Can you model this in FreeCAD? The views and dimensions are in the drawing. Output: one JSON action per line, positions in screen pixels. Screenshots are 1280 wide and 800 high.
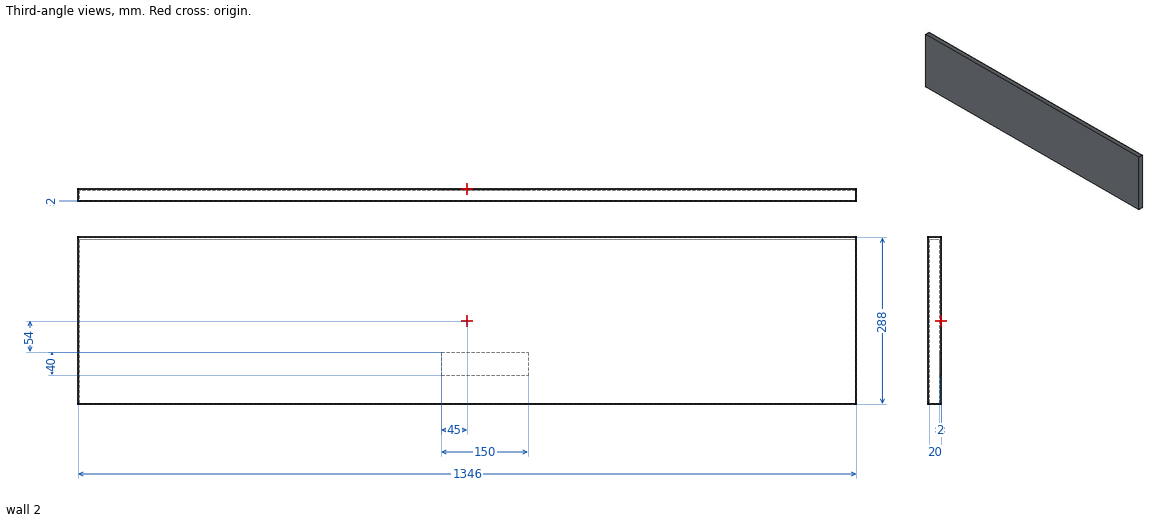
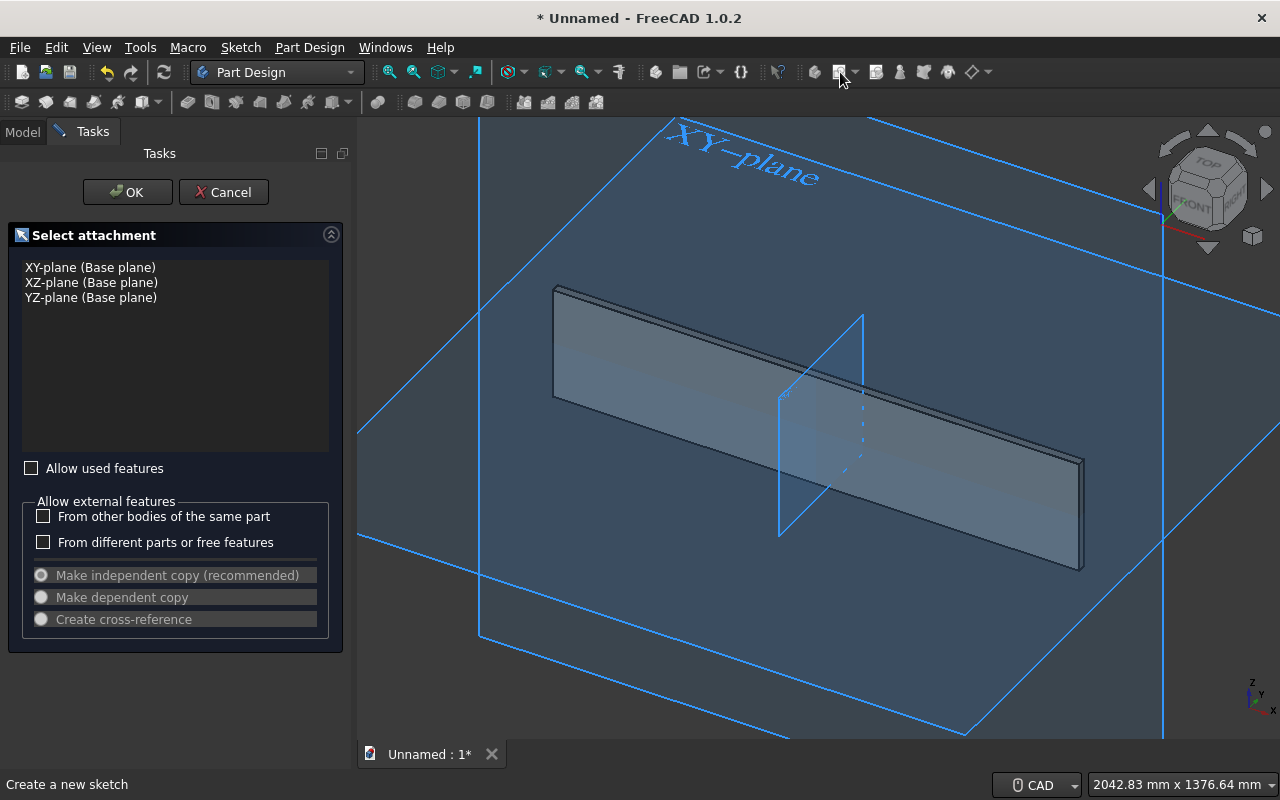
{"action": "left_click", "coordinate": [82, 282]}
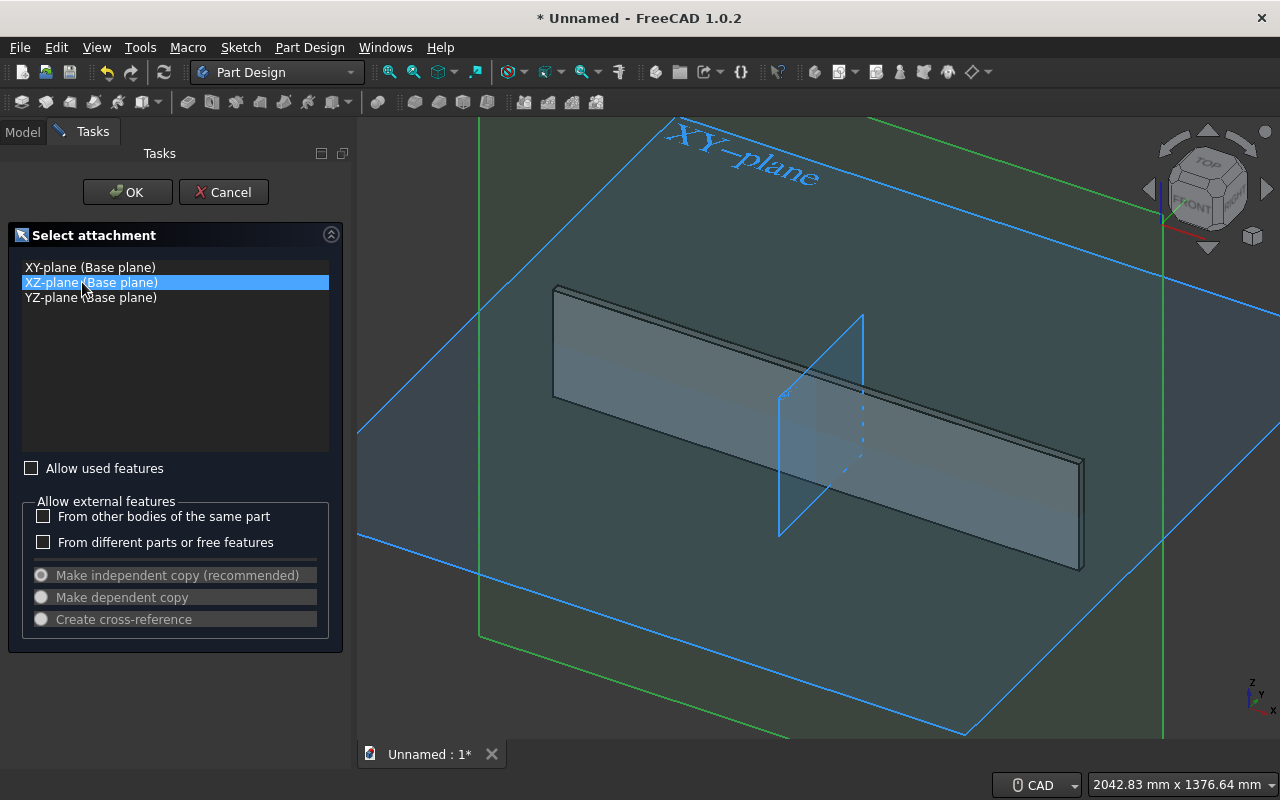
{"action": "left_click", "coordinate": [128, 192]}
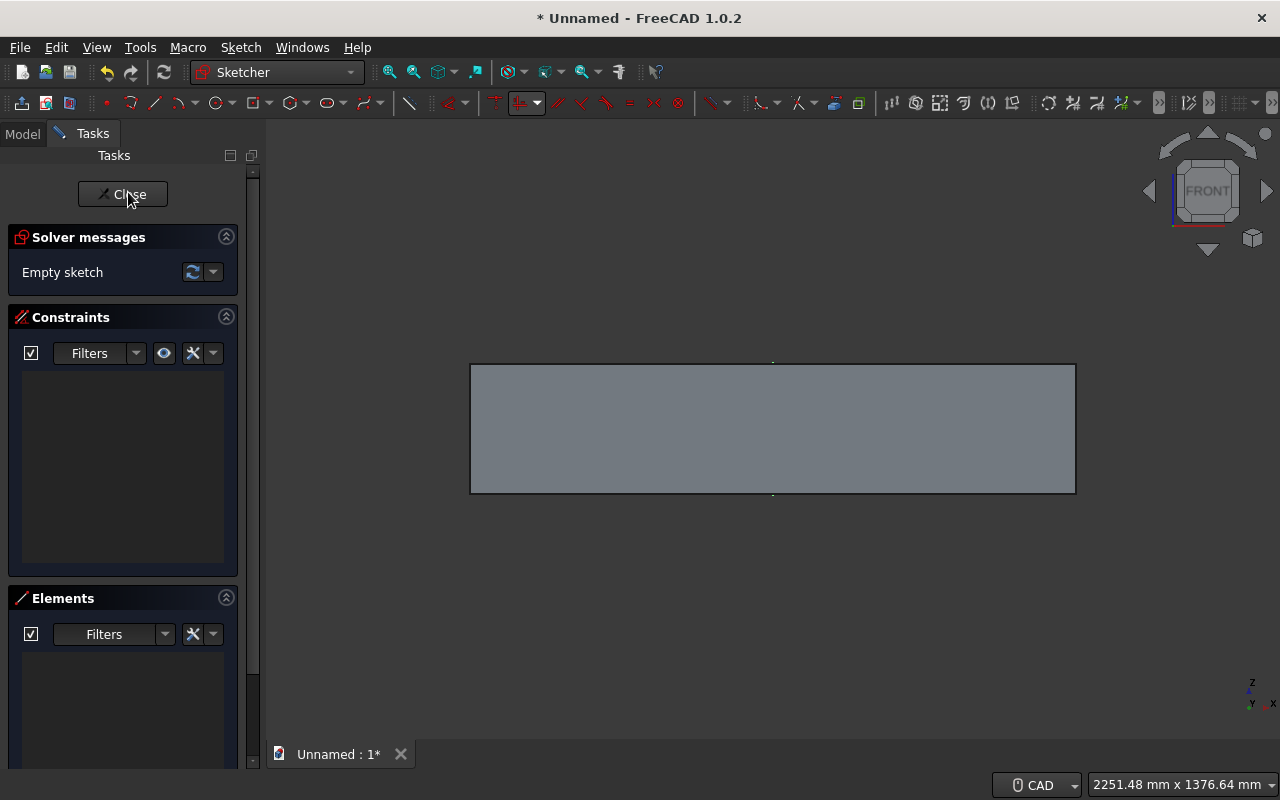
{"action": "key", "text": "q s"}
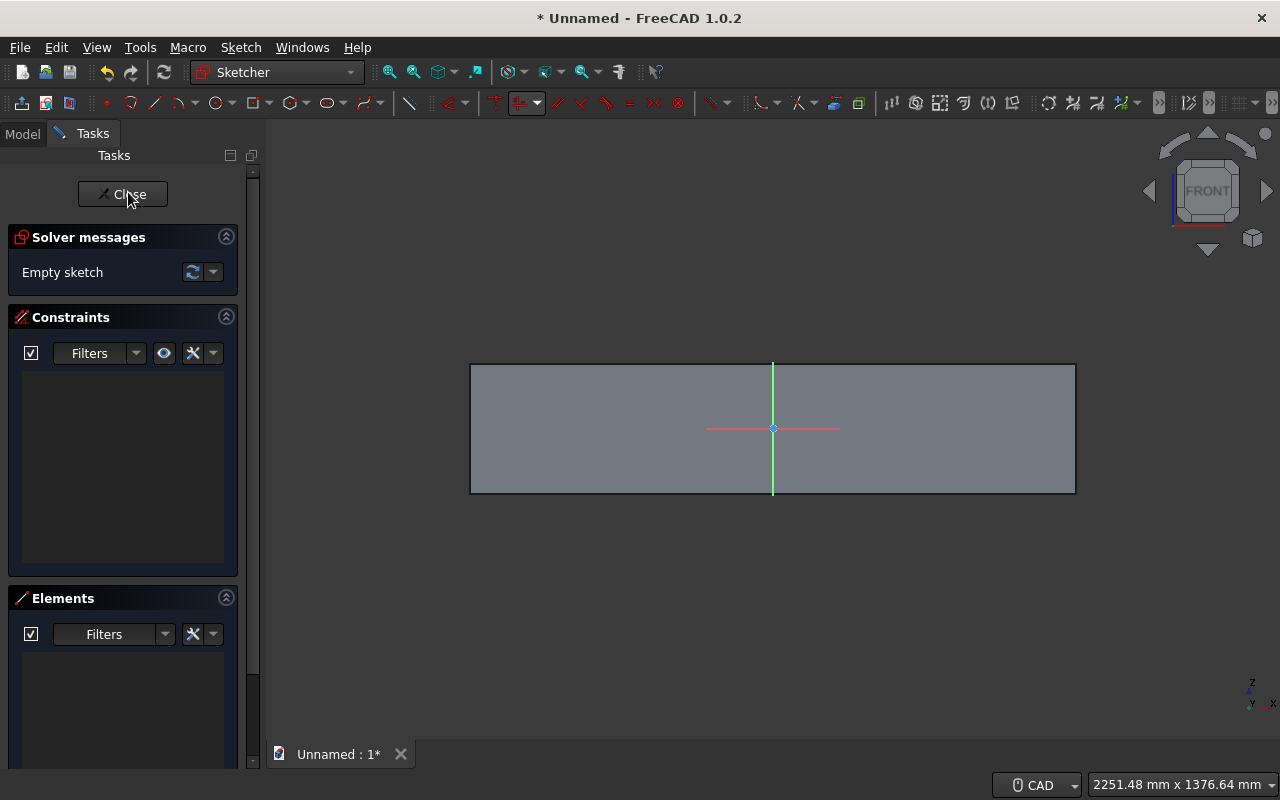
{"action": "scroll", "coordinate": [797, 453], "scroll_direction": "up", "scroll_amount": 11}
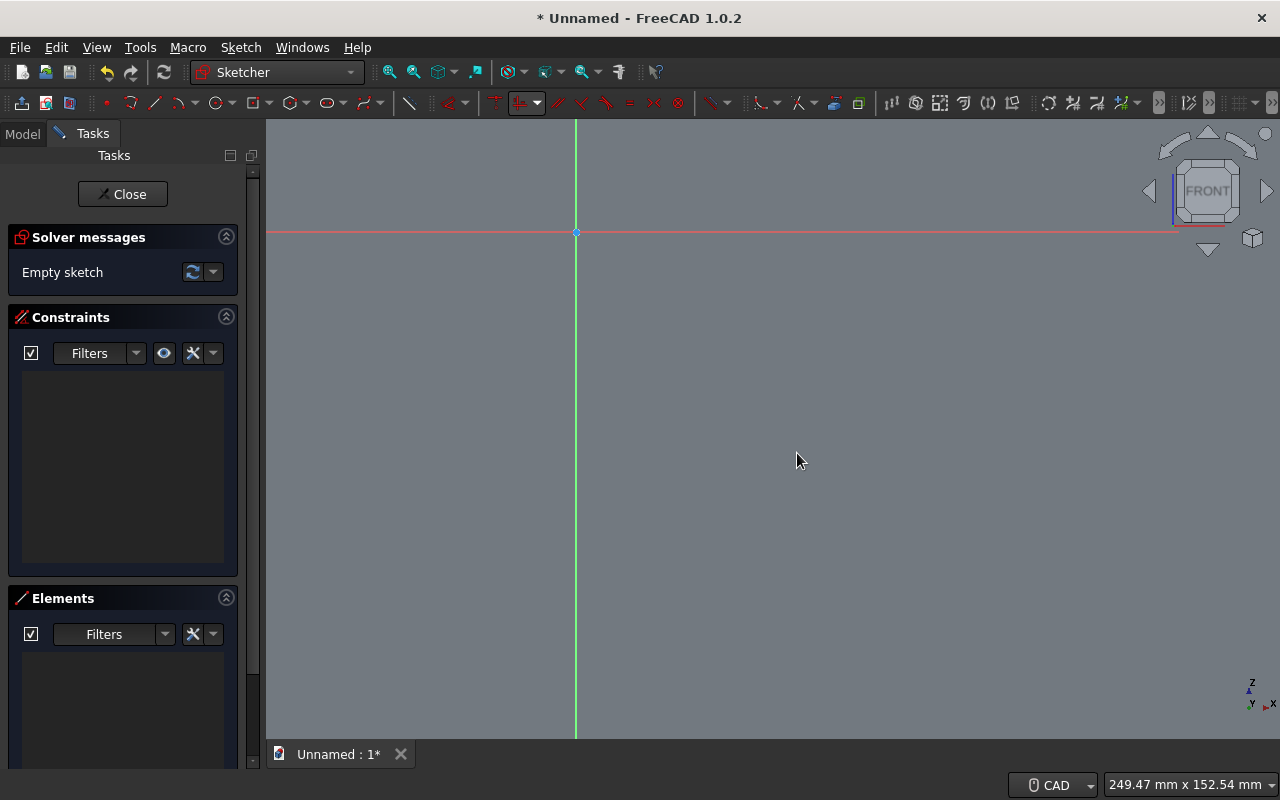
{"action": "key", "text": "g r"}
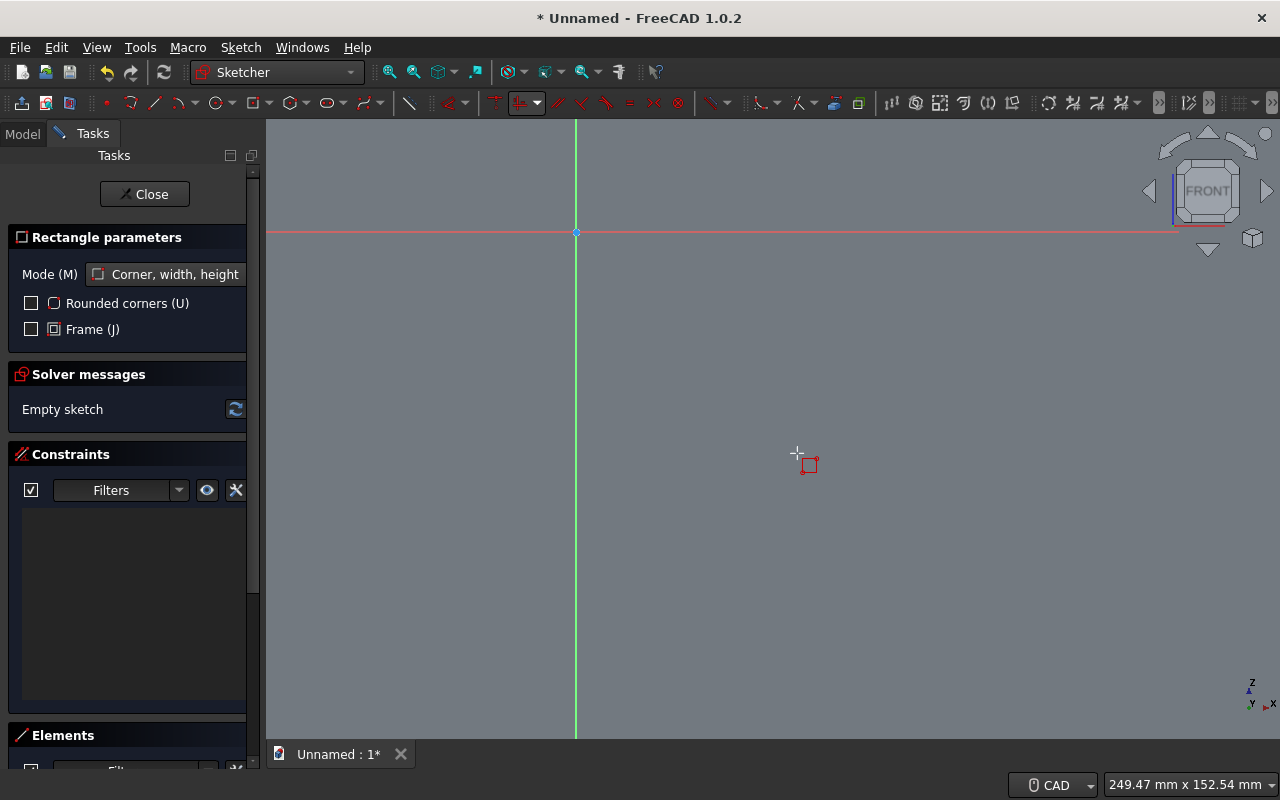
{"action": "left_click", "coordinate": [393, 452]}
{"action": "left_click", "coordinate": [1003, 614]}
{"action": "key", "text": "Escape"}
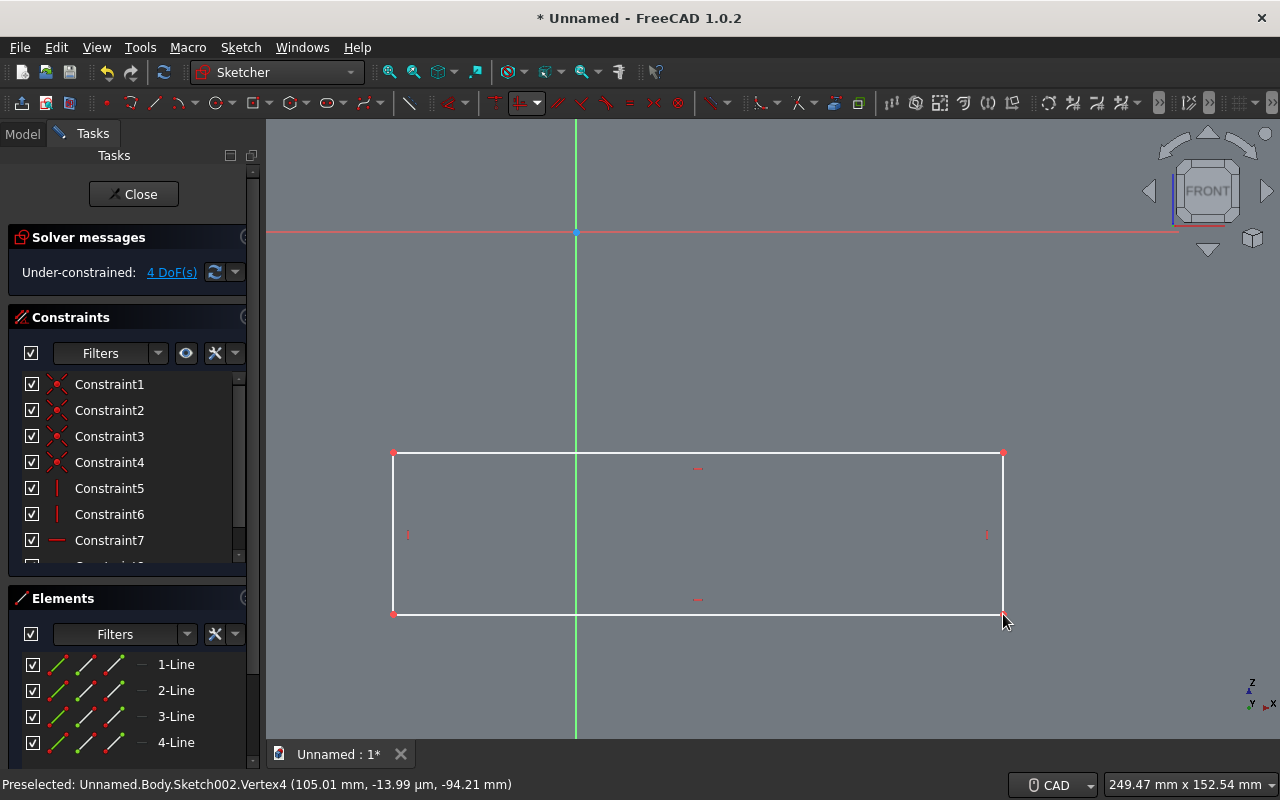
{"action": "left_click", "coordinate": [448, 104]}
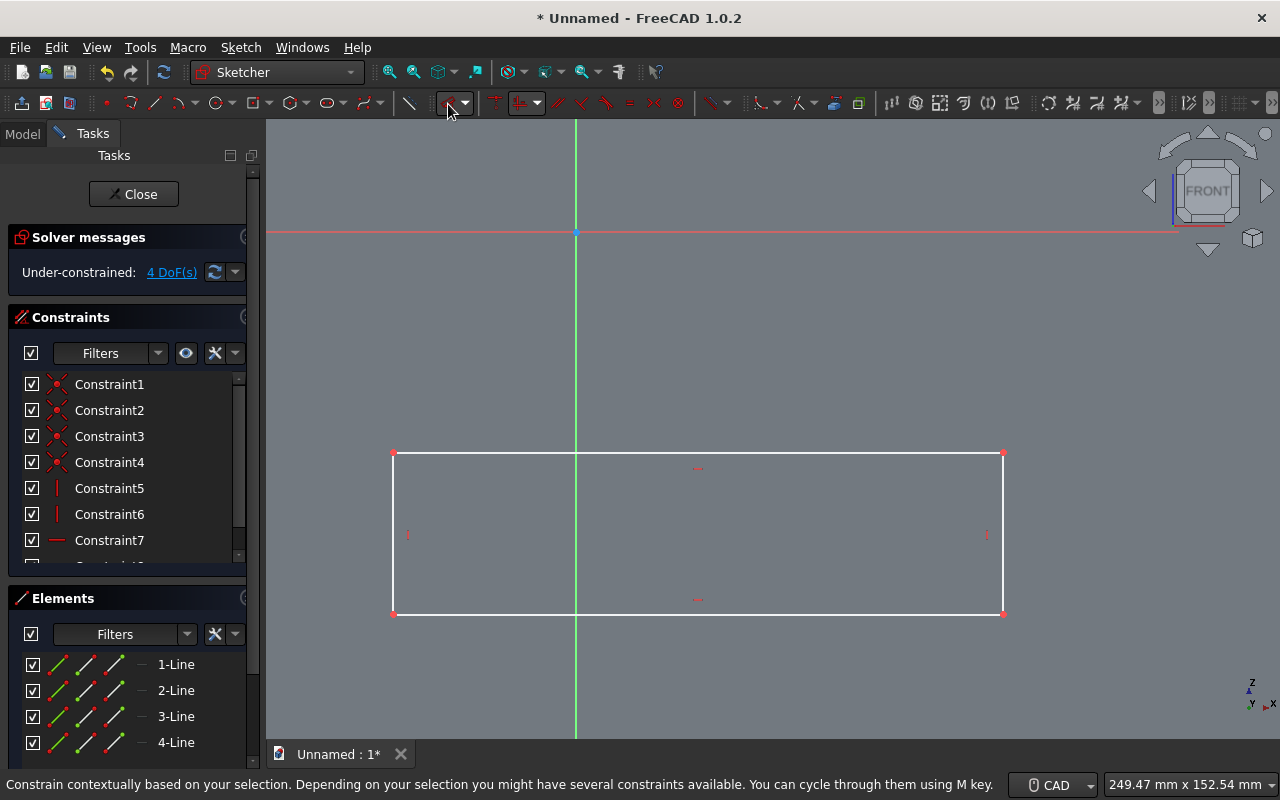
{"action": "left_click", "coordinate": [393, 502]}
{"action": "left_click", "coordinate": [359, 534]}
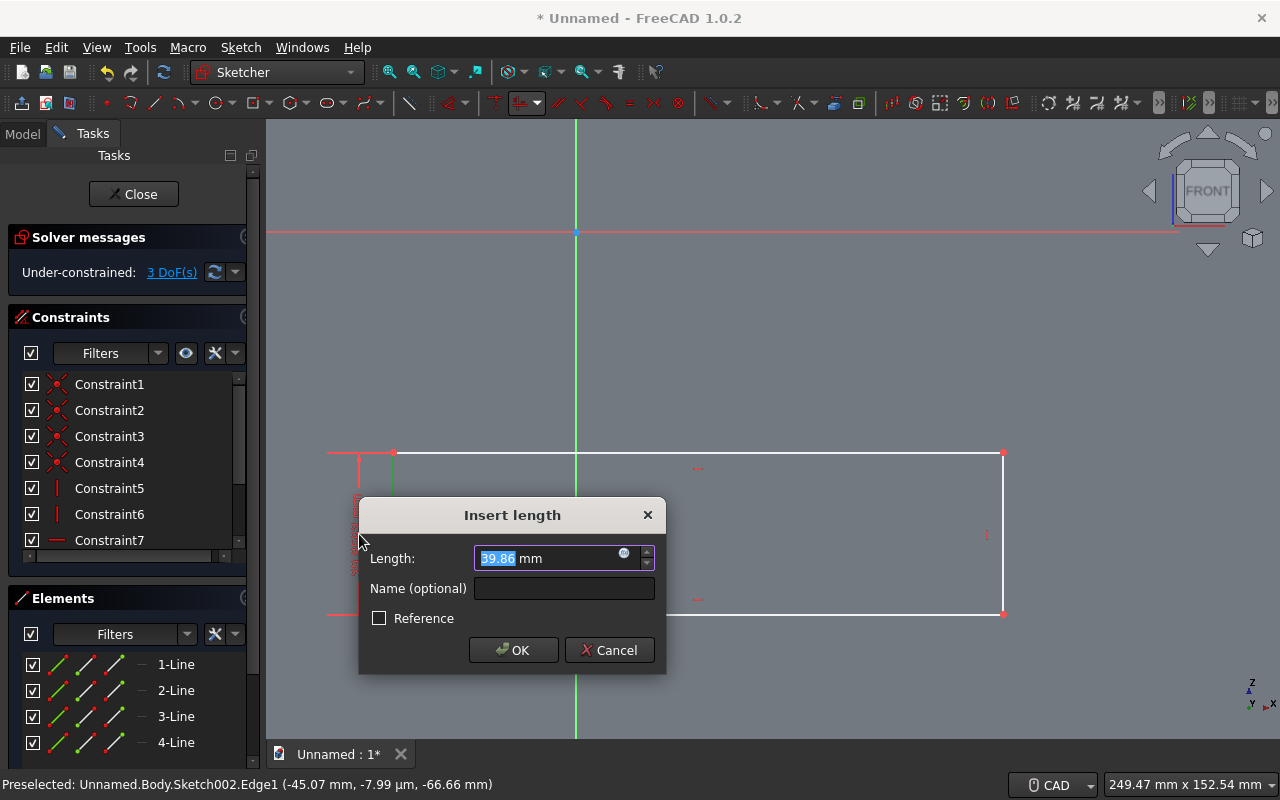
{"action": "type", "text": "40"}
{"action": "key", "text": "Return"}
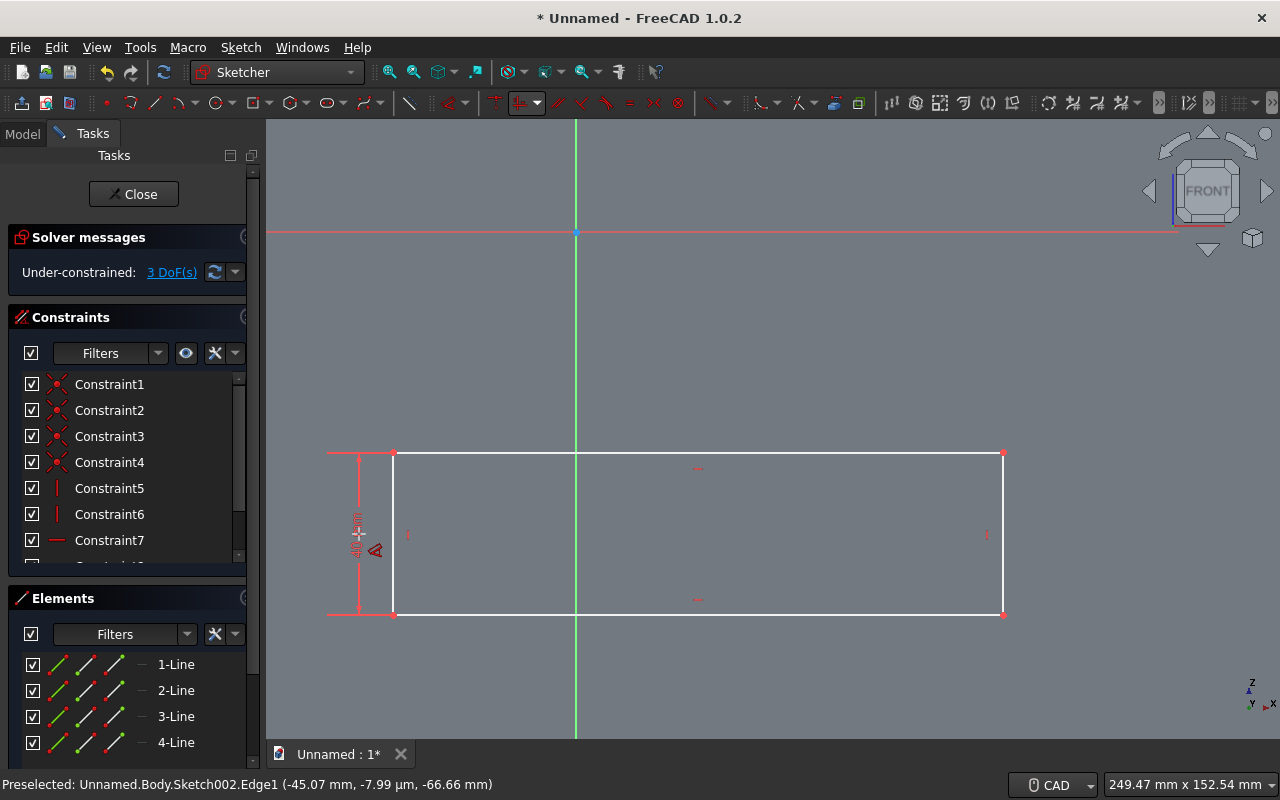
{"action": "left_click", "coordinate": [576, 615]}
{"action": "left_click", "coordinate": [698, 649]}